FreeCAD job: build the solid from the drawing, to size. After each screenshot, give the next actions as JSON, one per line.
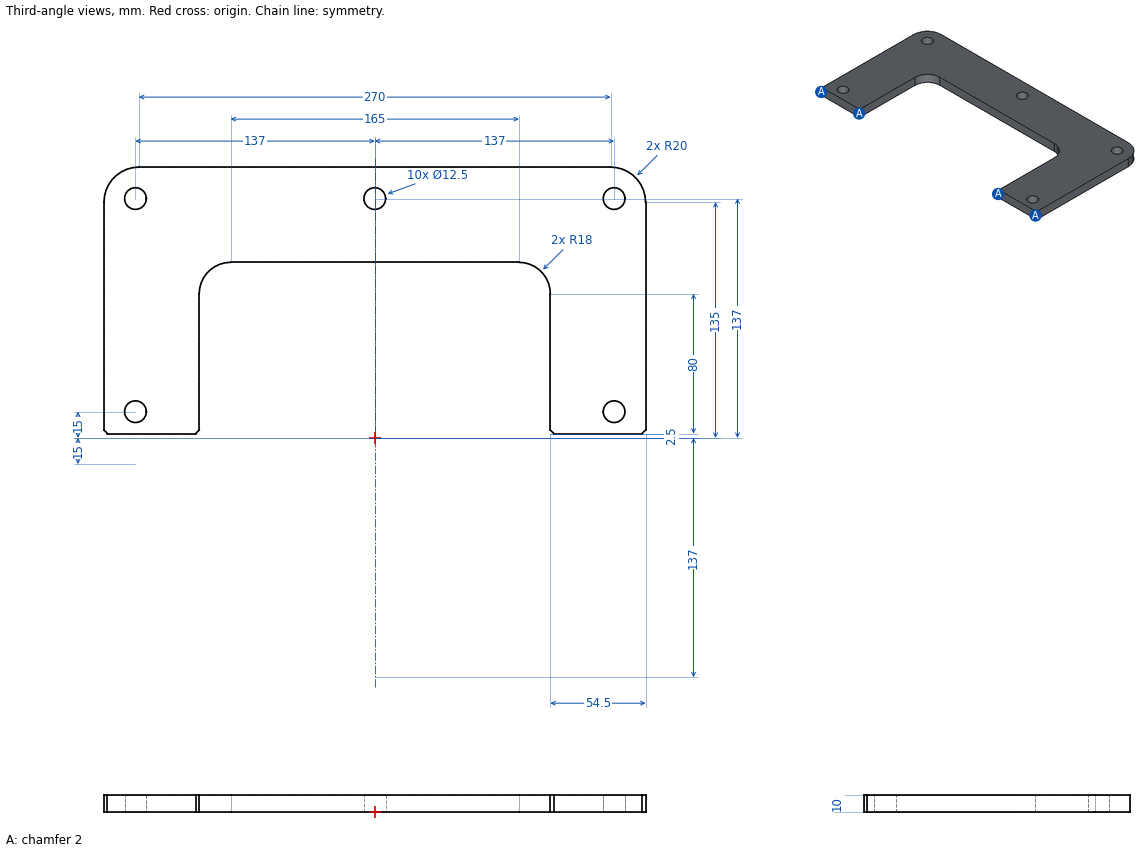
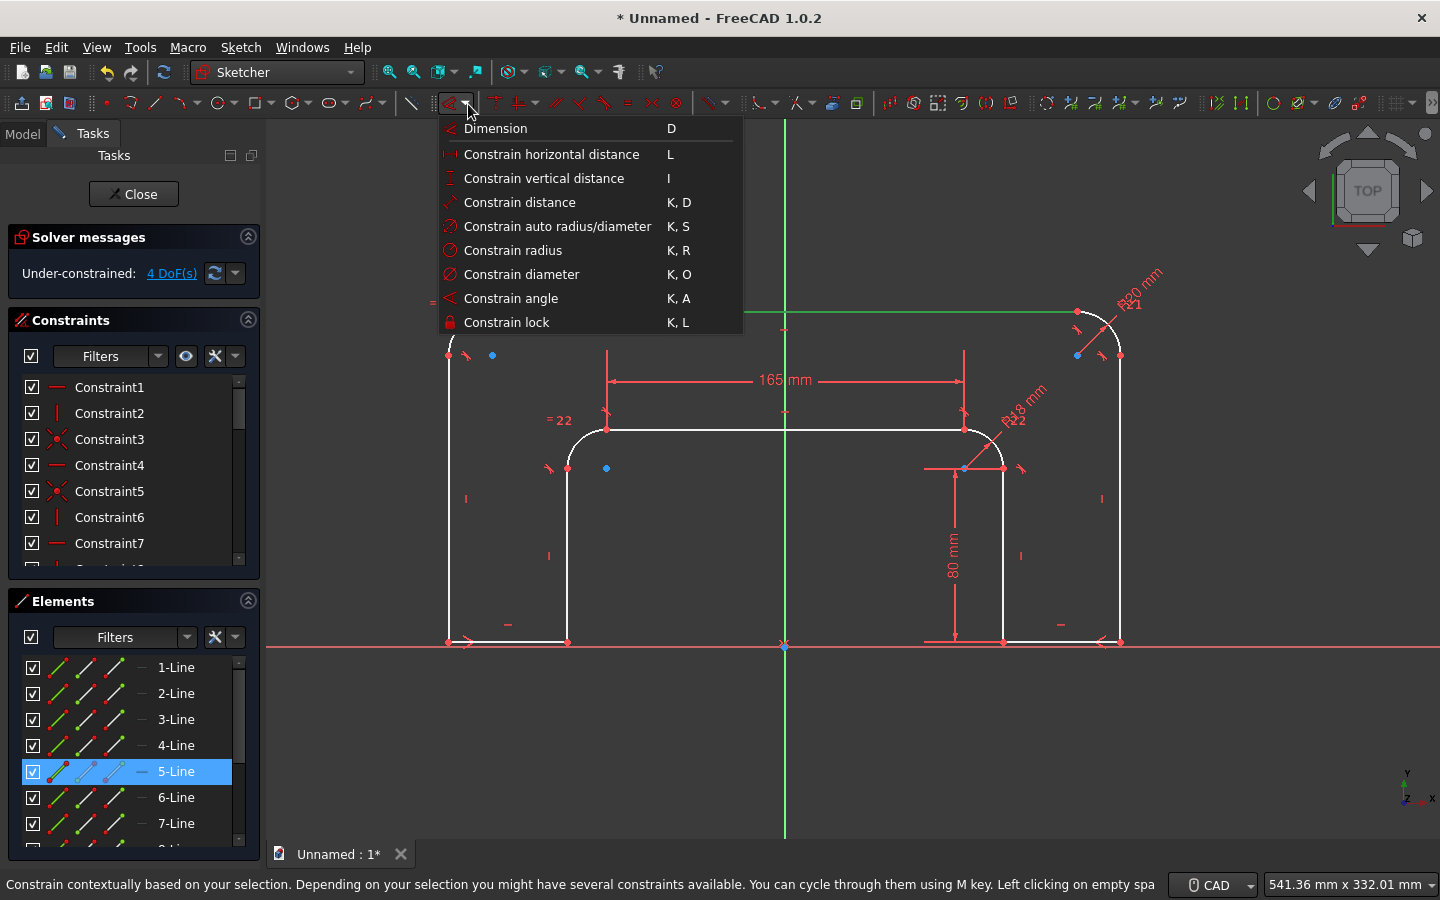
{"action": "left_click", "coordinate": [591, 154]}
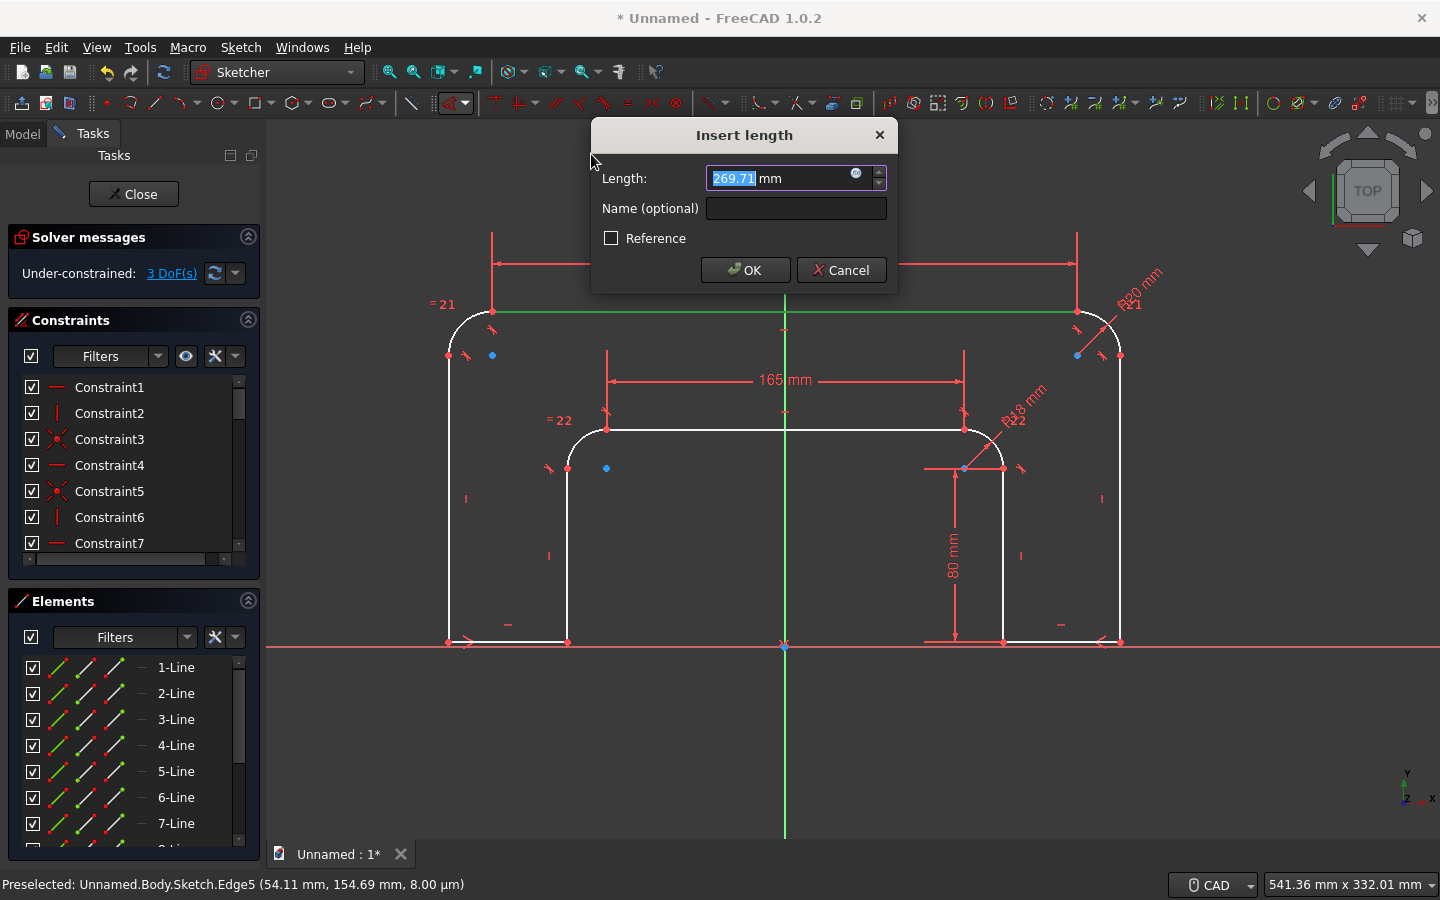
{"action": "type", "text": "270"}
{"action": "key", "text": "Return"}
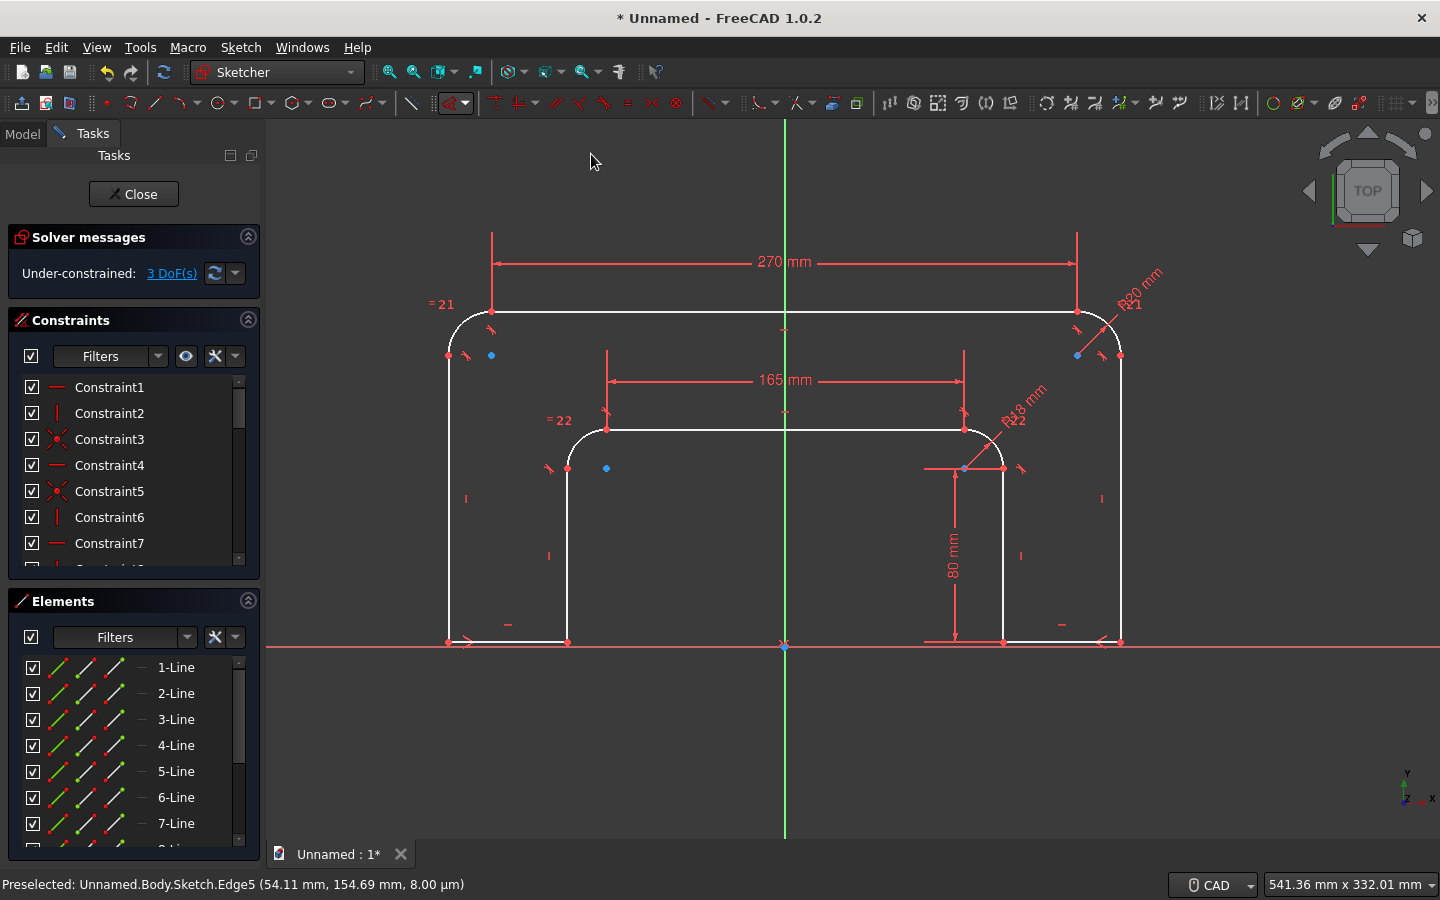
{"action": "scroll", "coordinate": [1039, 642], "scroll_direction": "up", "scroll_amount": 6}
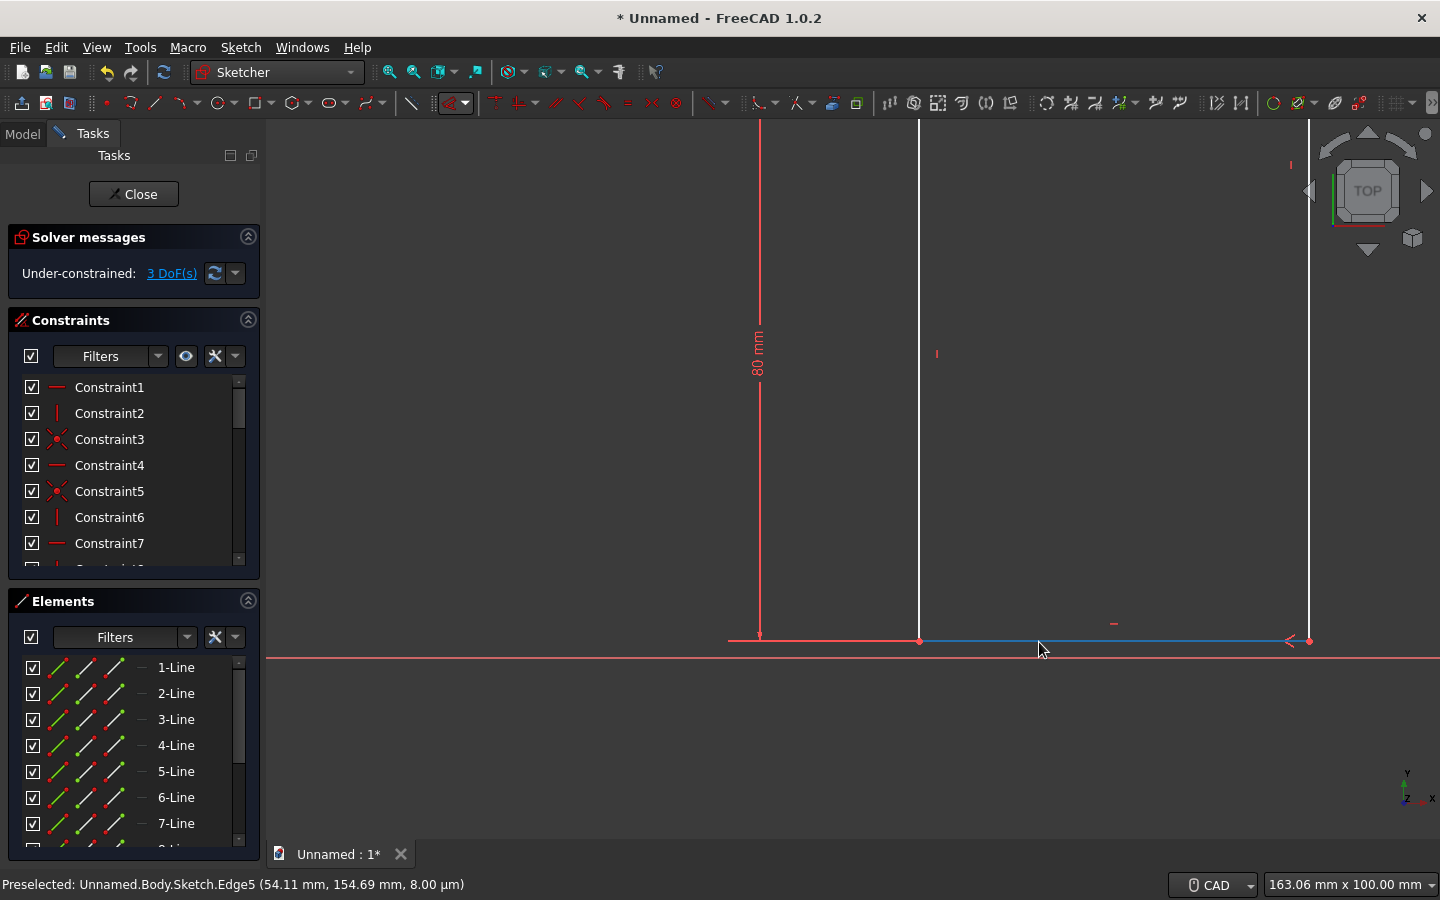
{"action": "left_click", "coordinate": [1036, 641]}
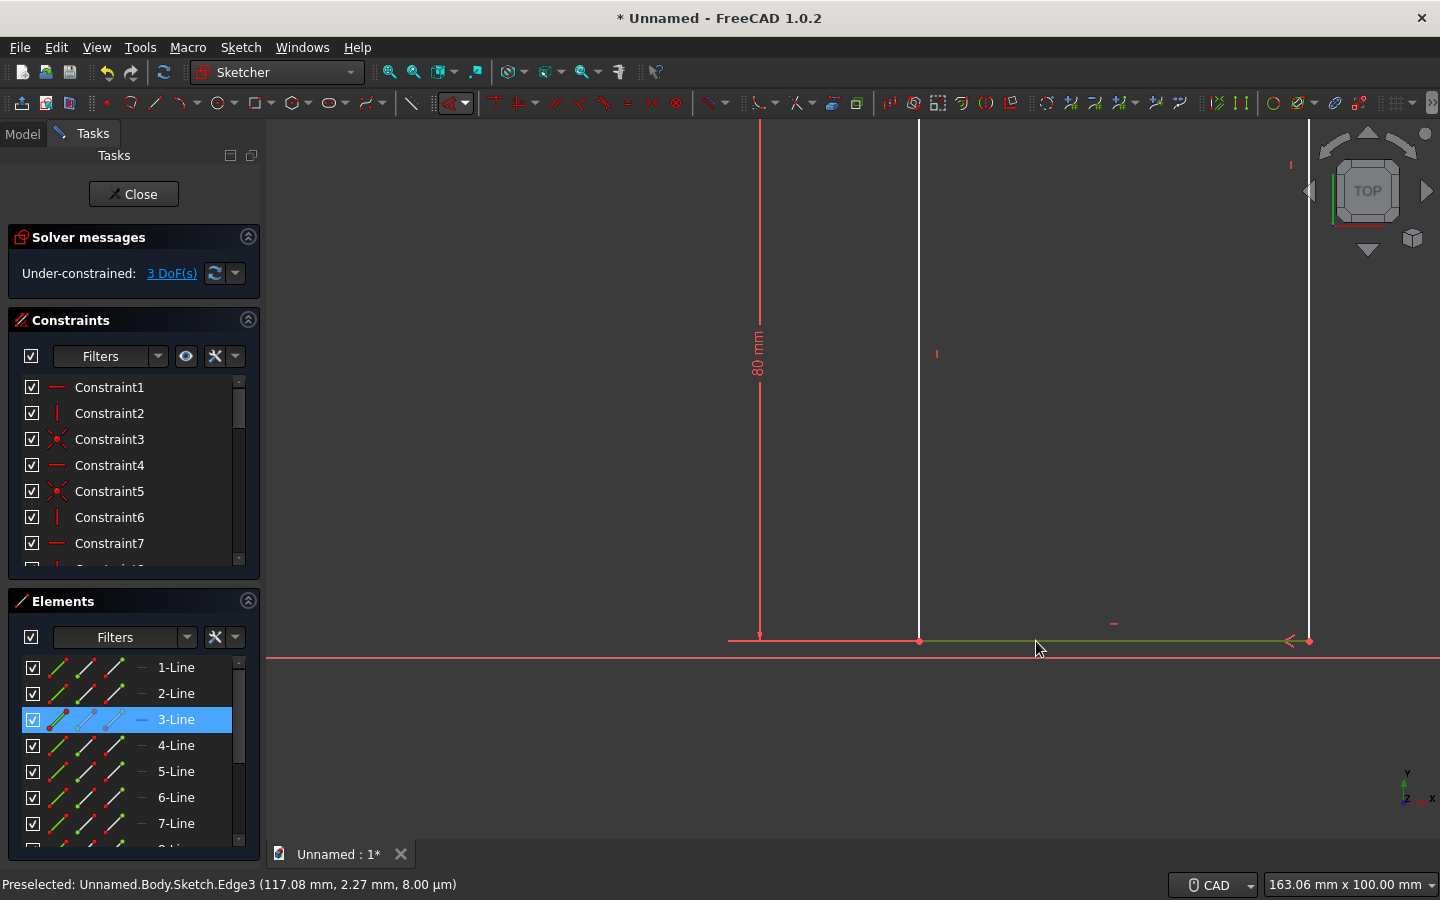
{"action": "key", "text": "l"}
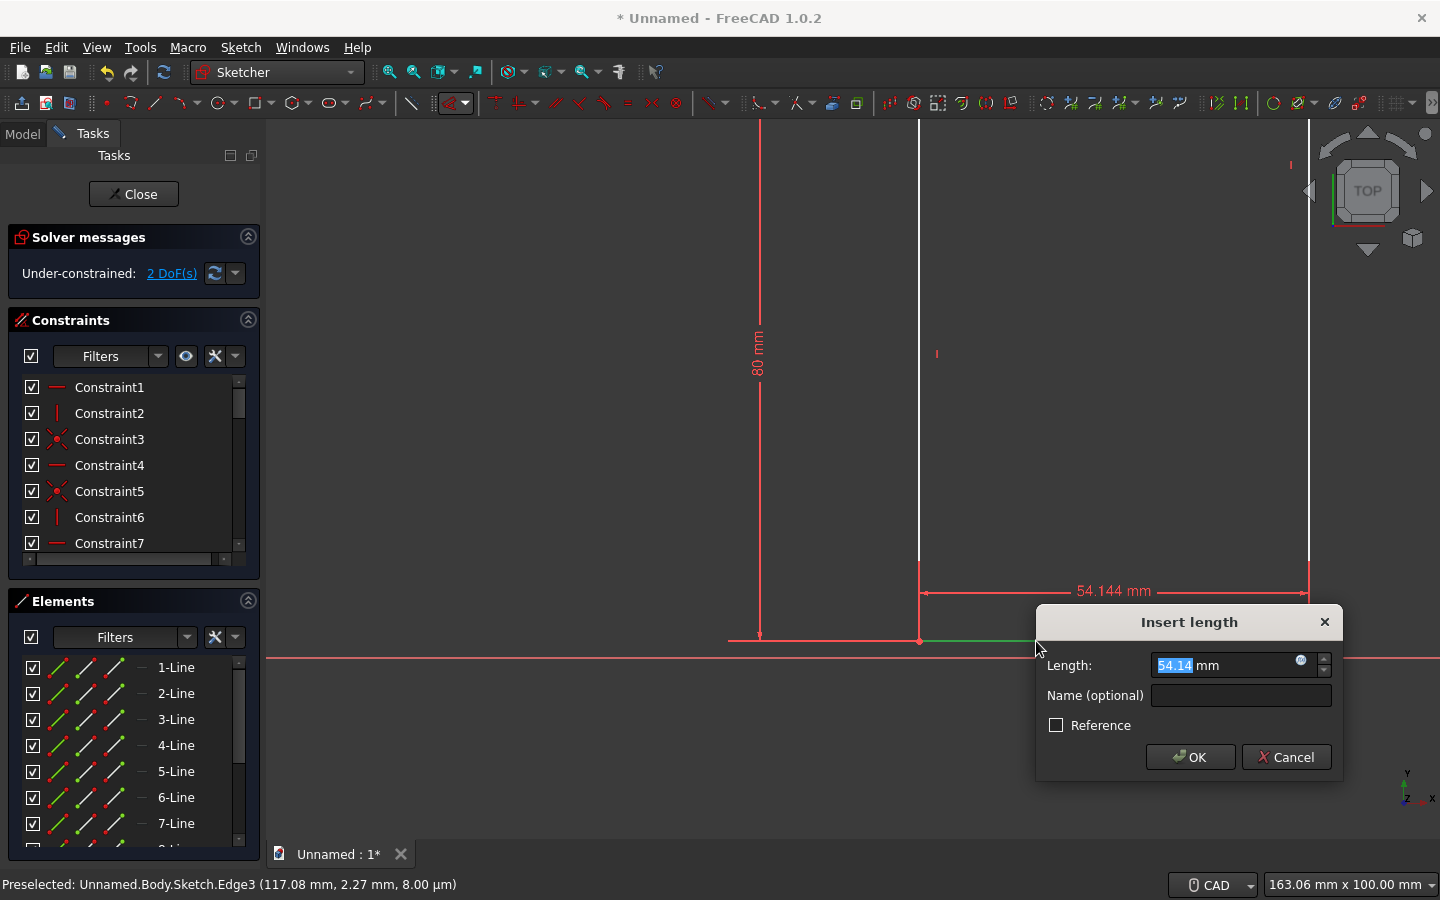
{"action": "type", "text": "54.5"}
{"action": "key", "text": "Return"}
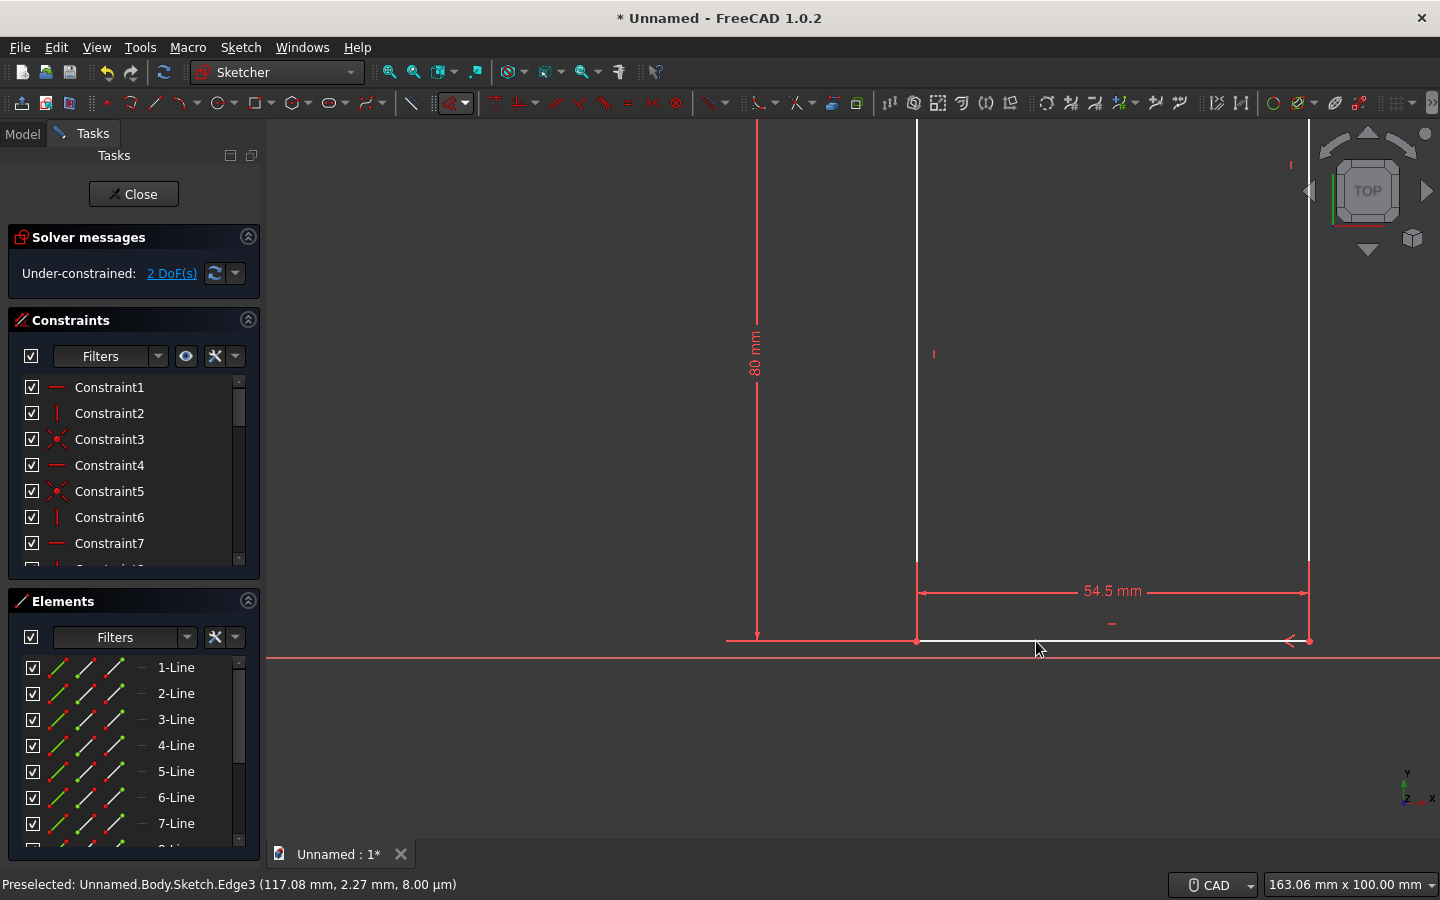
{"action": "scroll", "coordinate": [917, 641], "scroll_direction": "up", "scroll_amount": 4}